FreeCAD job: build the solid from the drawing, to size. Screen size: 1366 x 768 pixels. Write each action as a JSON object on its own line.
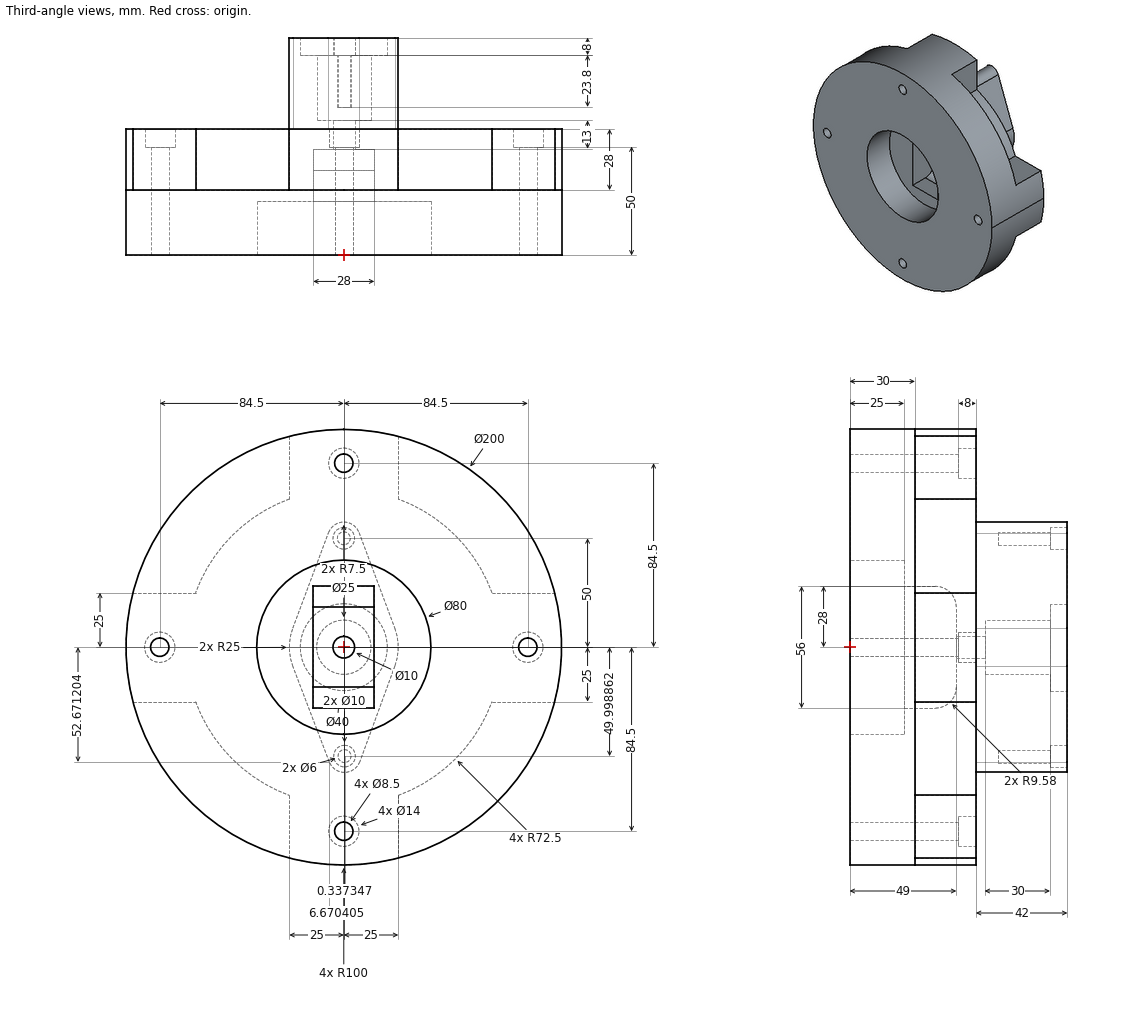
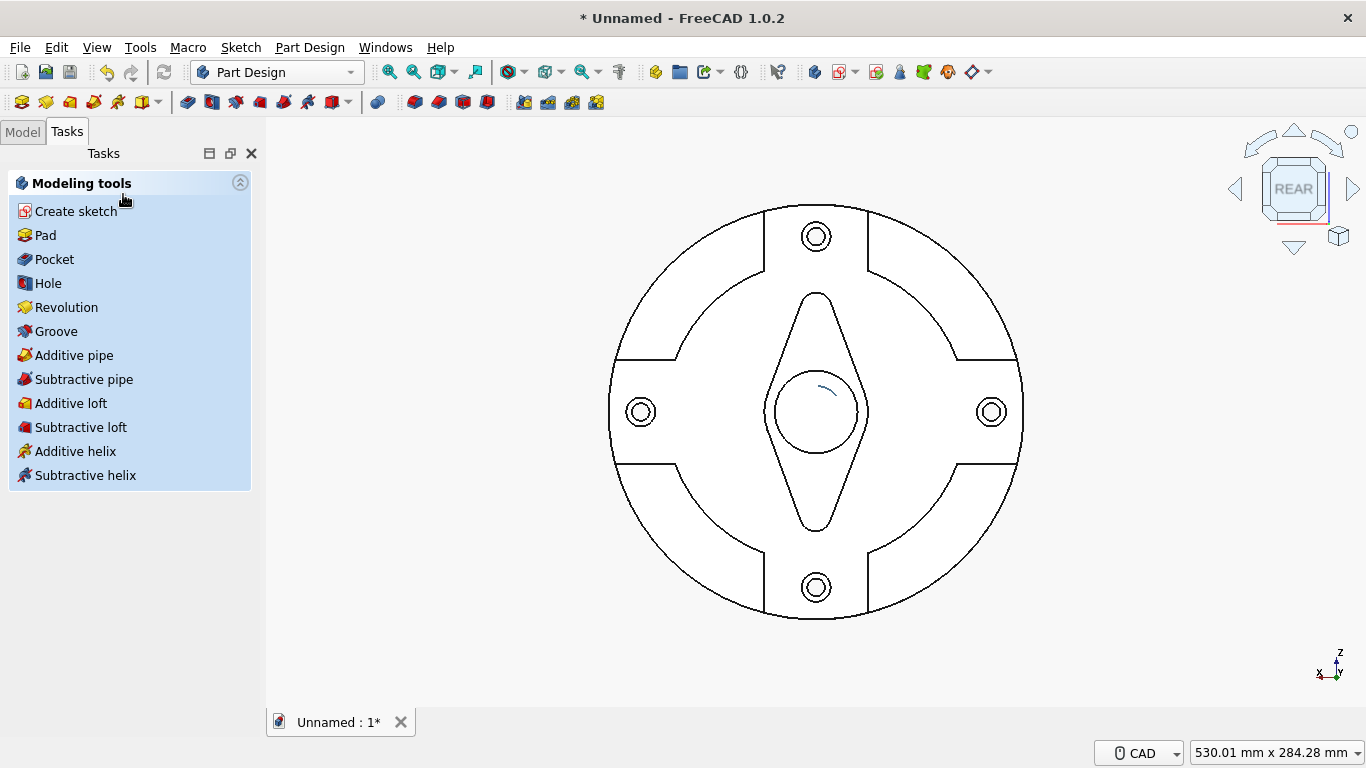
{"action": "left_click", "coordinate": [188, 102]}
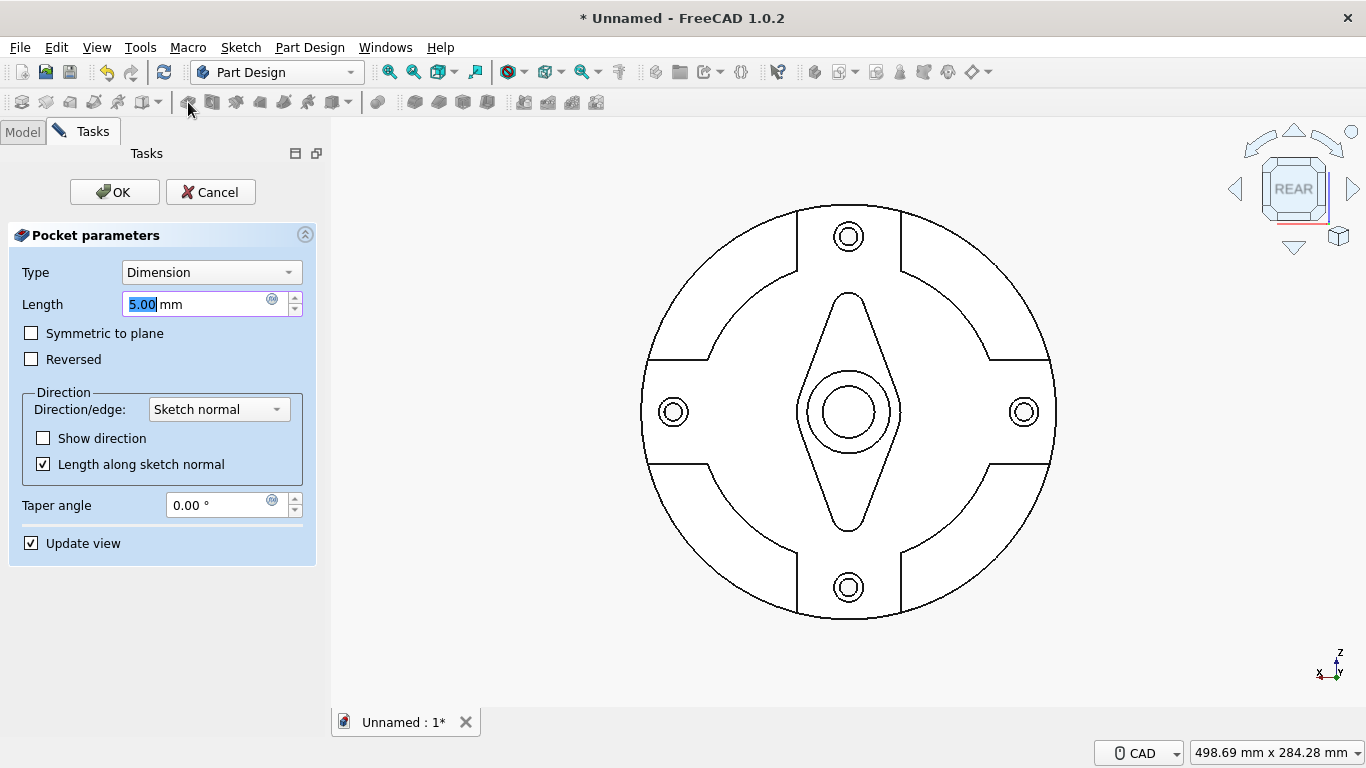
{"action": "type", "text": "30"}
{"action": "key", "text": "Tab"}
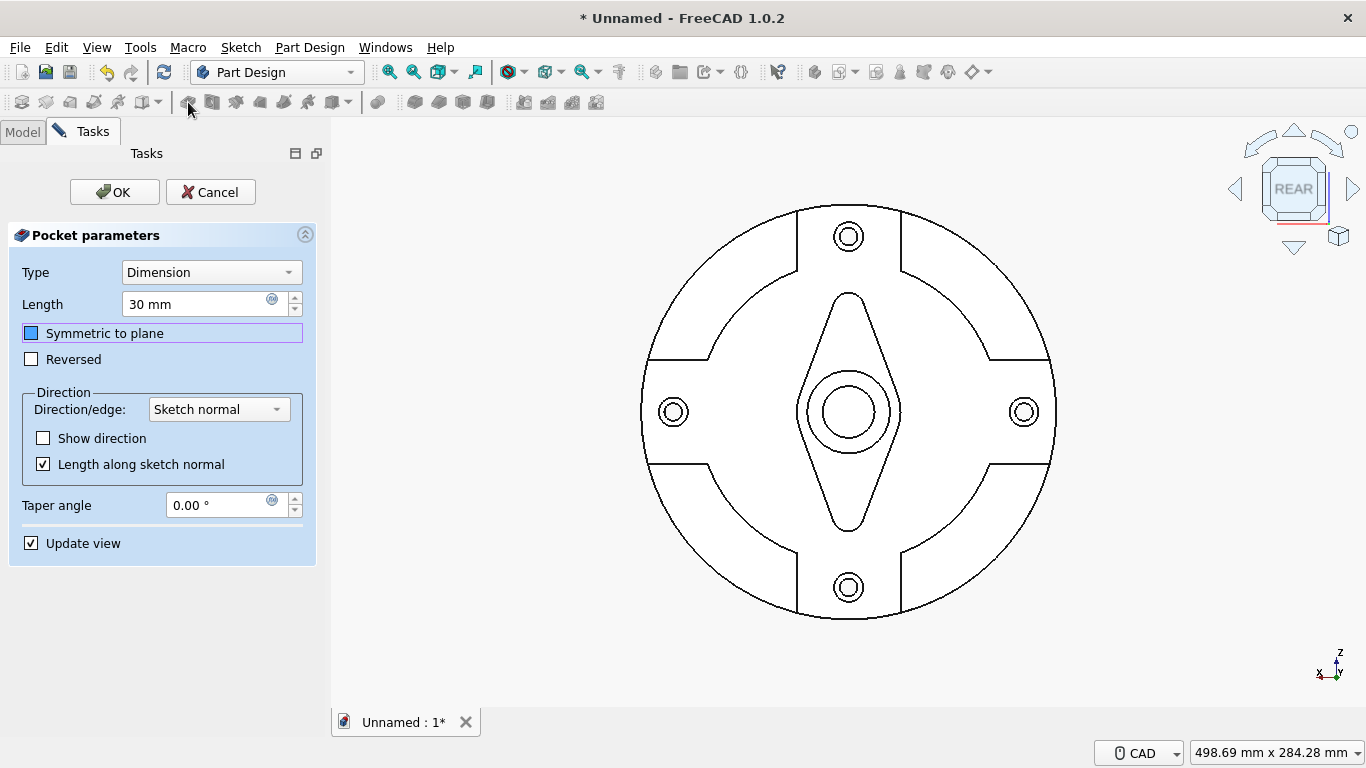
{"action": "left_click", "coordinate": [115, 192]}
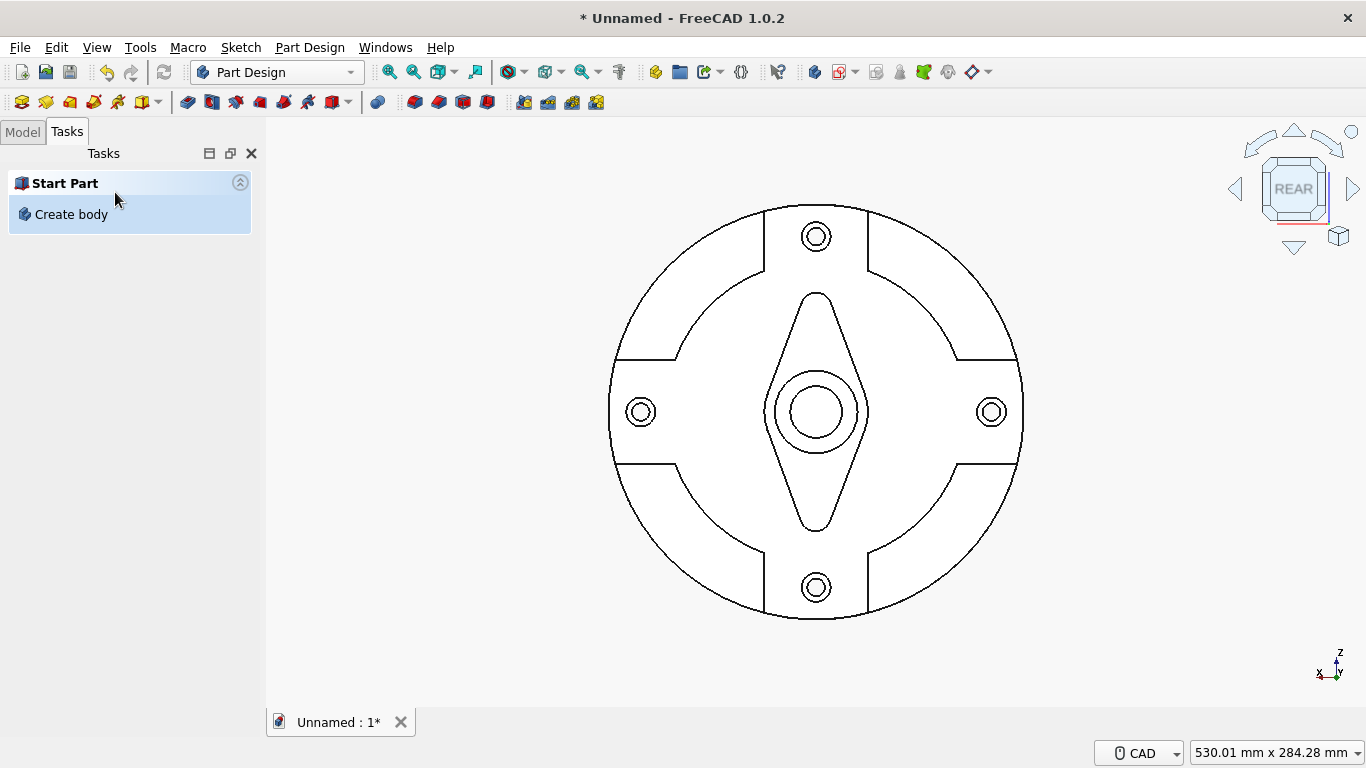
{"action": "left_click", "coordinate": [816, 411]}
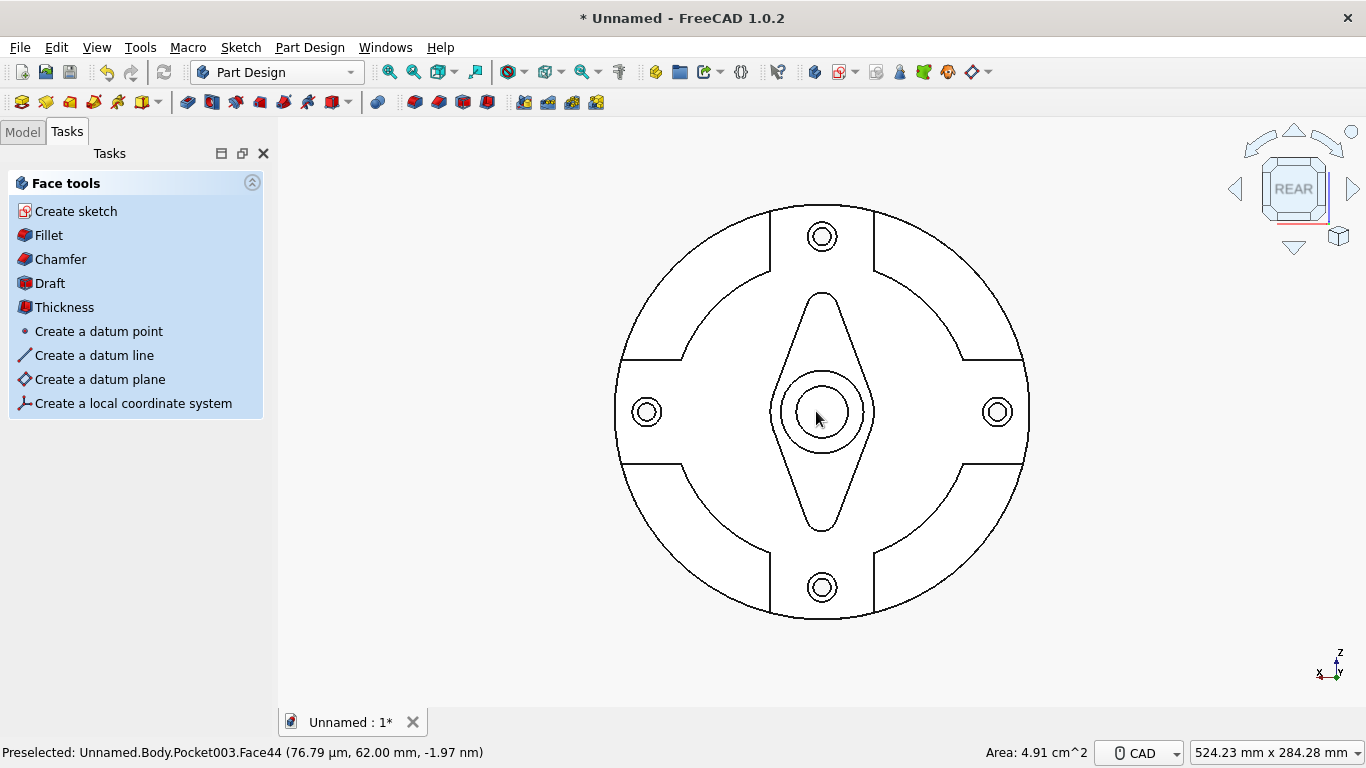
{"action": "left_click", "coordinate": [840, 72]}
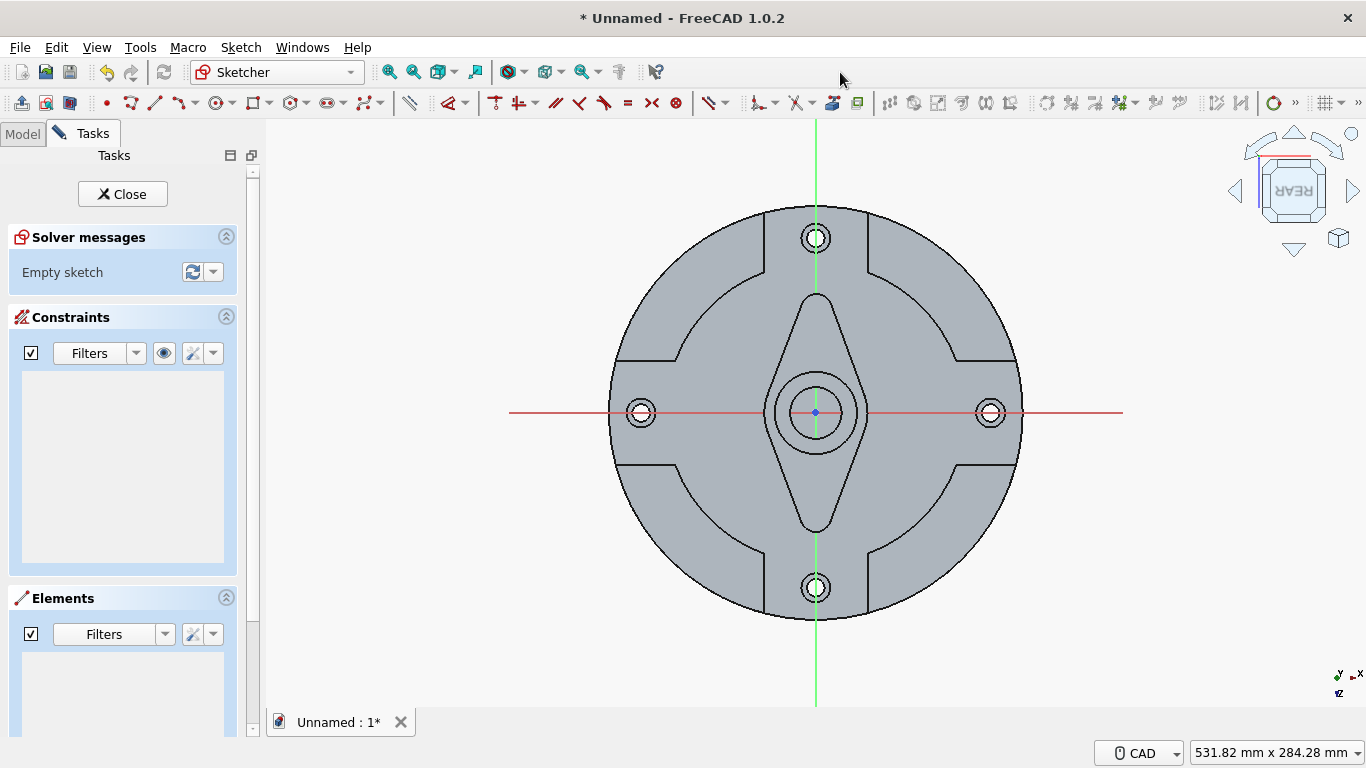
{"action": "left_click", "coordinate": [70, 104]}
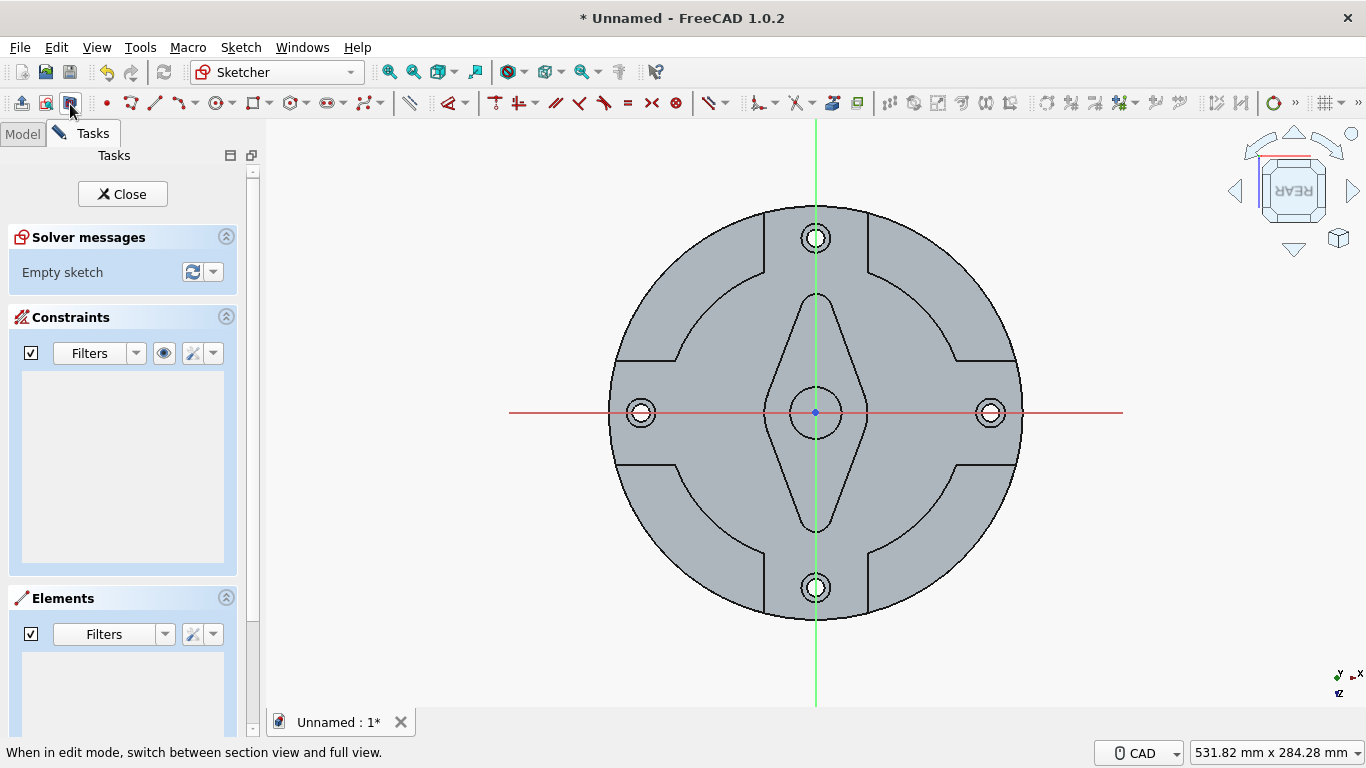
{"action": "scroll", "coordinate": [820, 413], "scroll_direction": "up", "scroll_amount": 14}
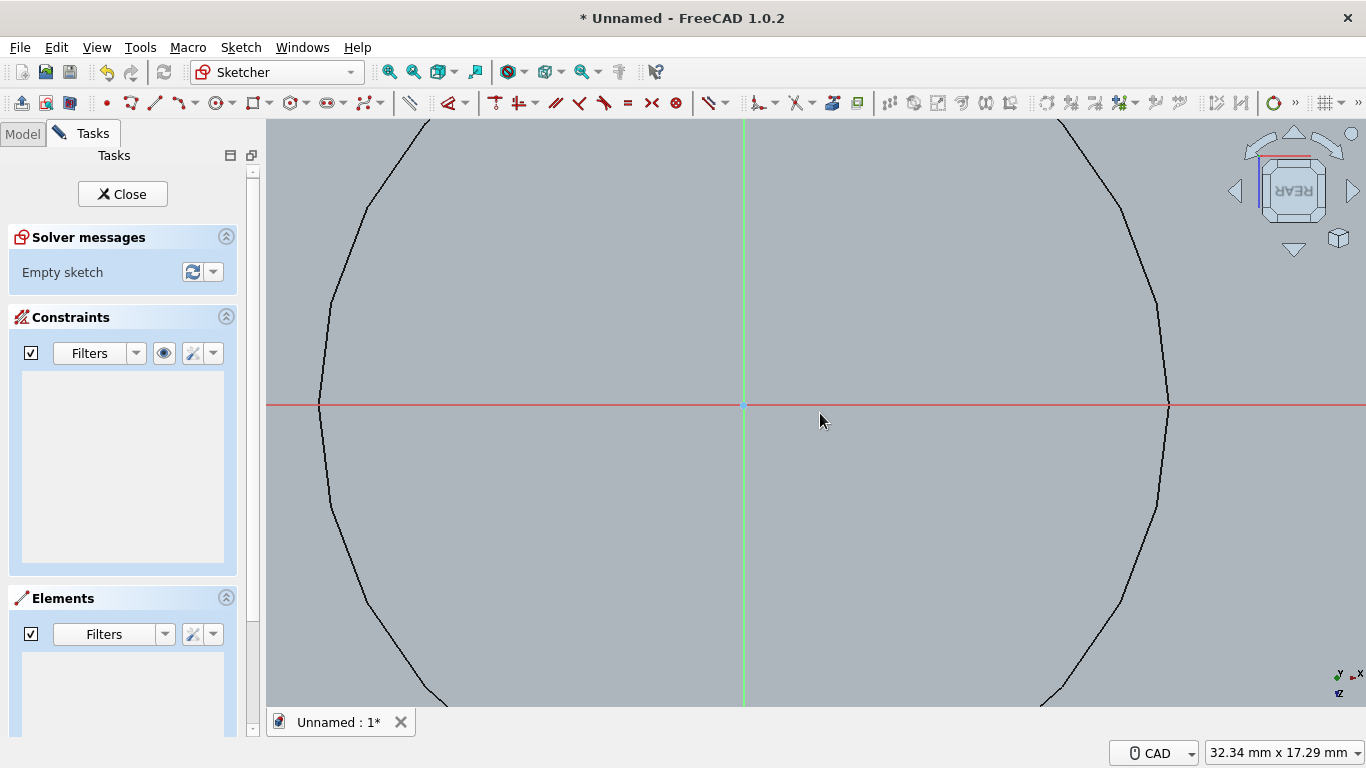
{"action": "key", "text": "g c"}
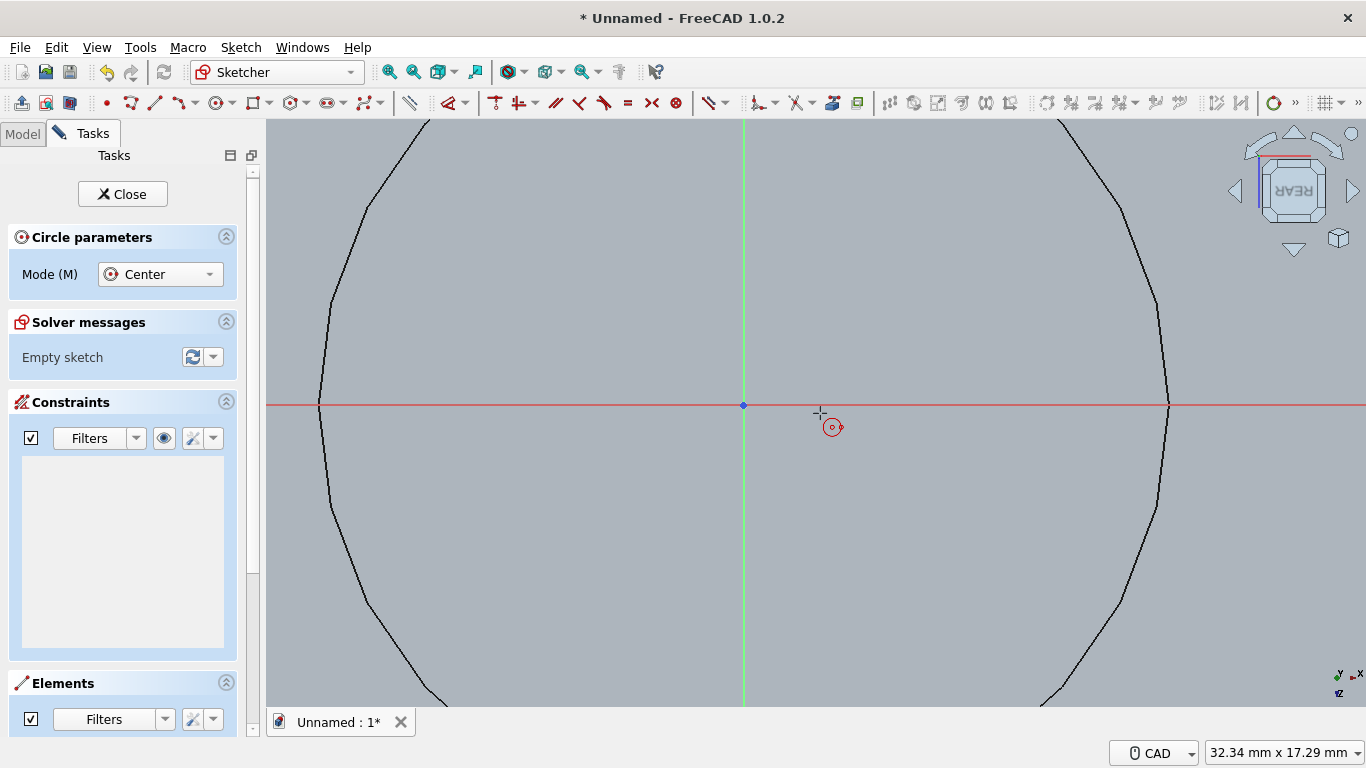
{"action": "left_click", "coordinate": [744, 405]}
{"action": "left_click", "coordinate": [864, 285]}
{"action": "key", "text": "Escape"}